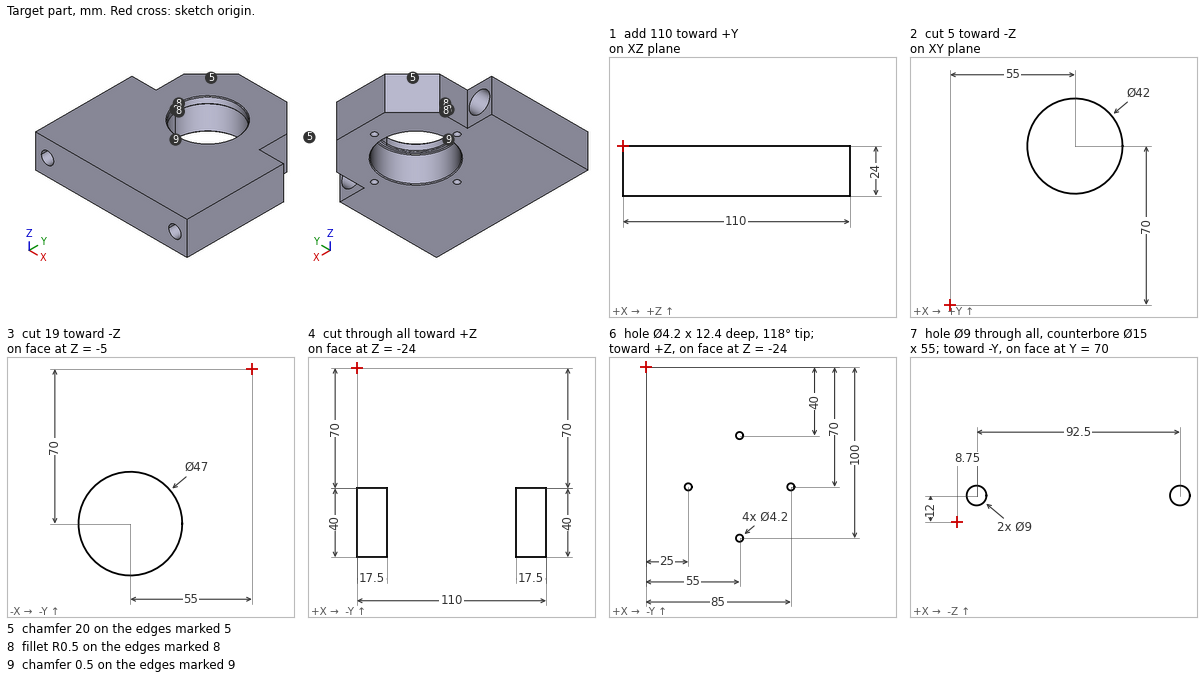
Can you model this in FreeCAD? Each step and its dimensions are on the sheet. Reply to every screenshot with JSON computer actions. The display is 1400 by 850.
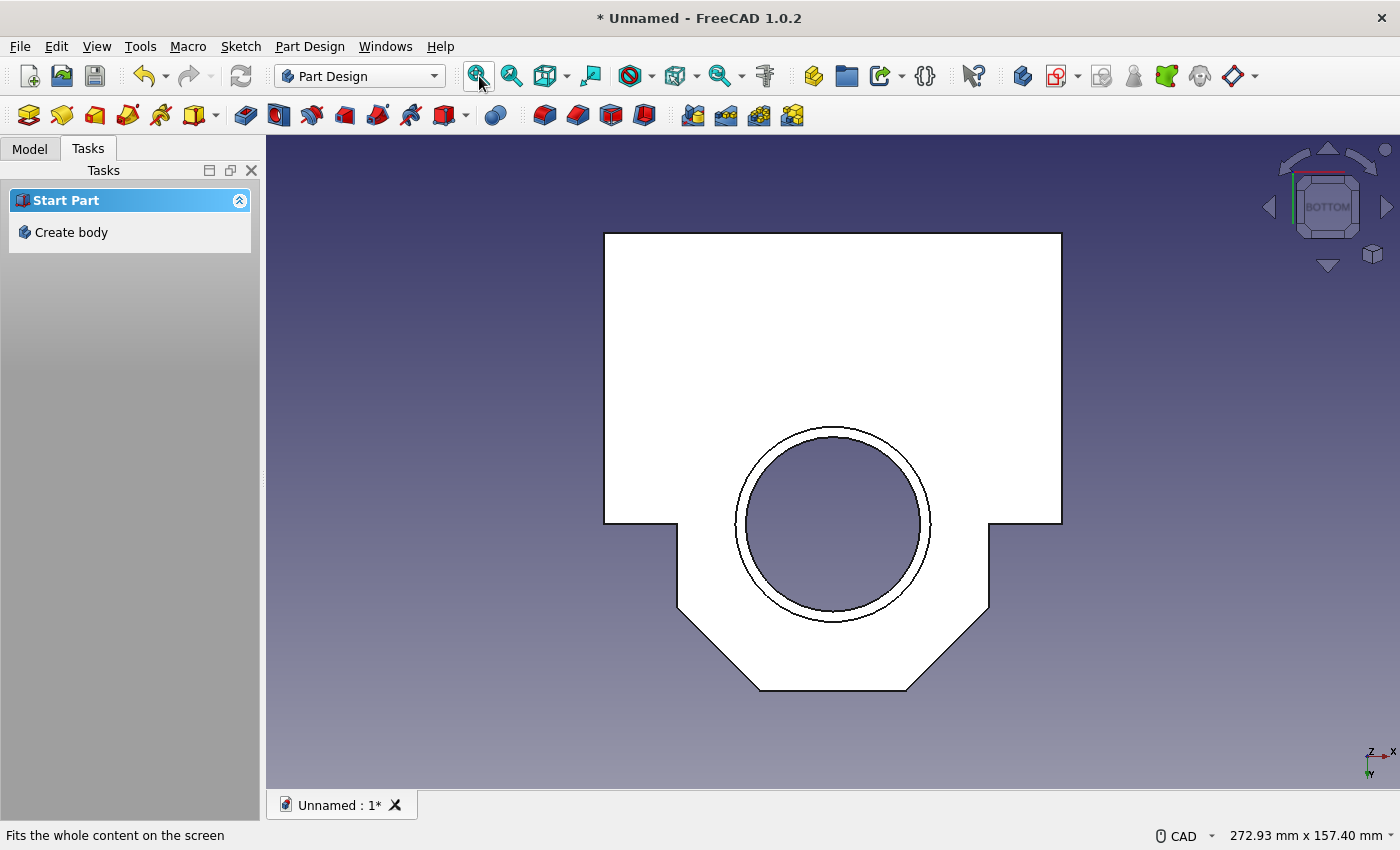
{"action": "left_click", "coordinate": [898, 330]}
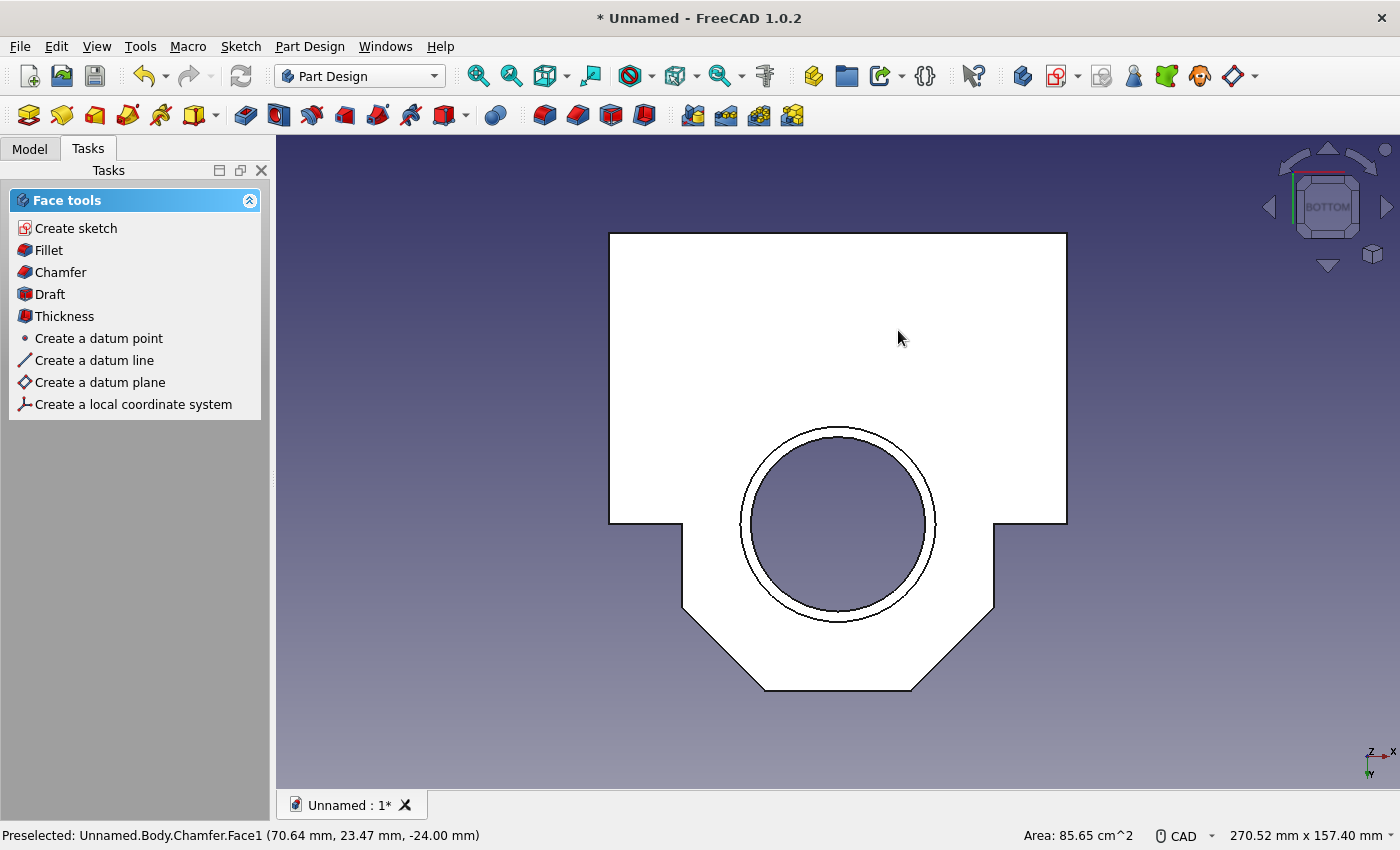
{"action": "left_click", "coordinate": [1056, 76]}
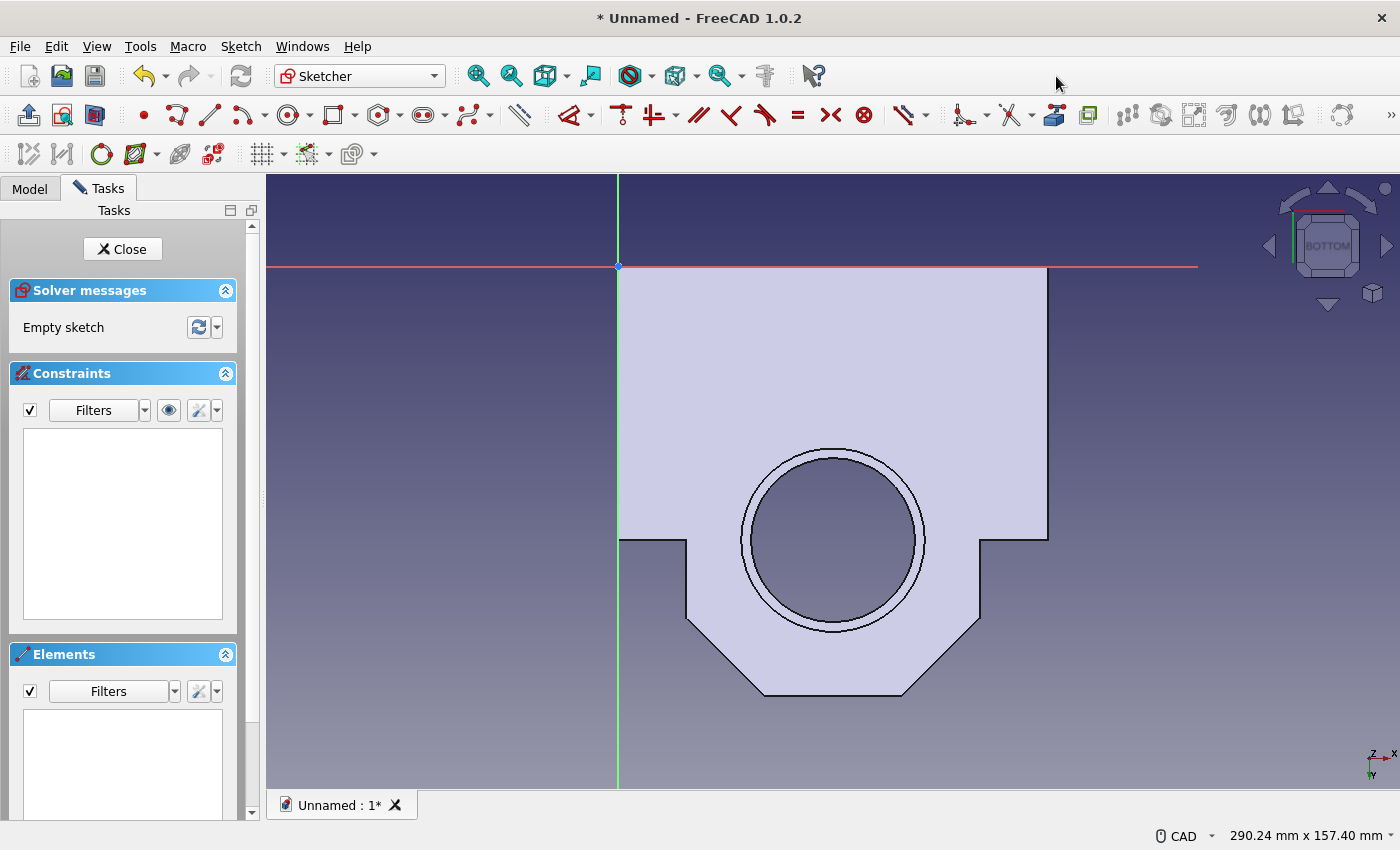
{"action": "left_click", "coordinate": [288, 116]}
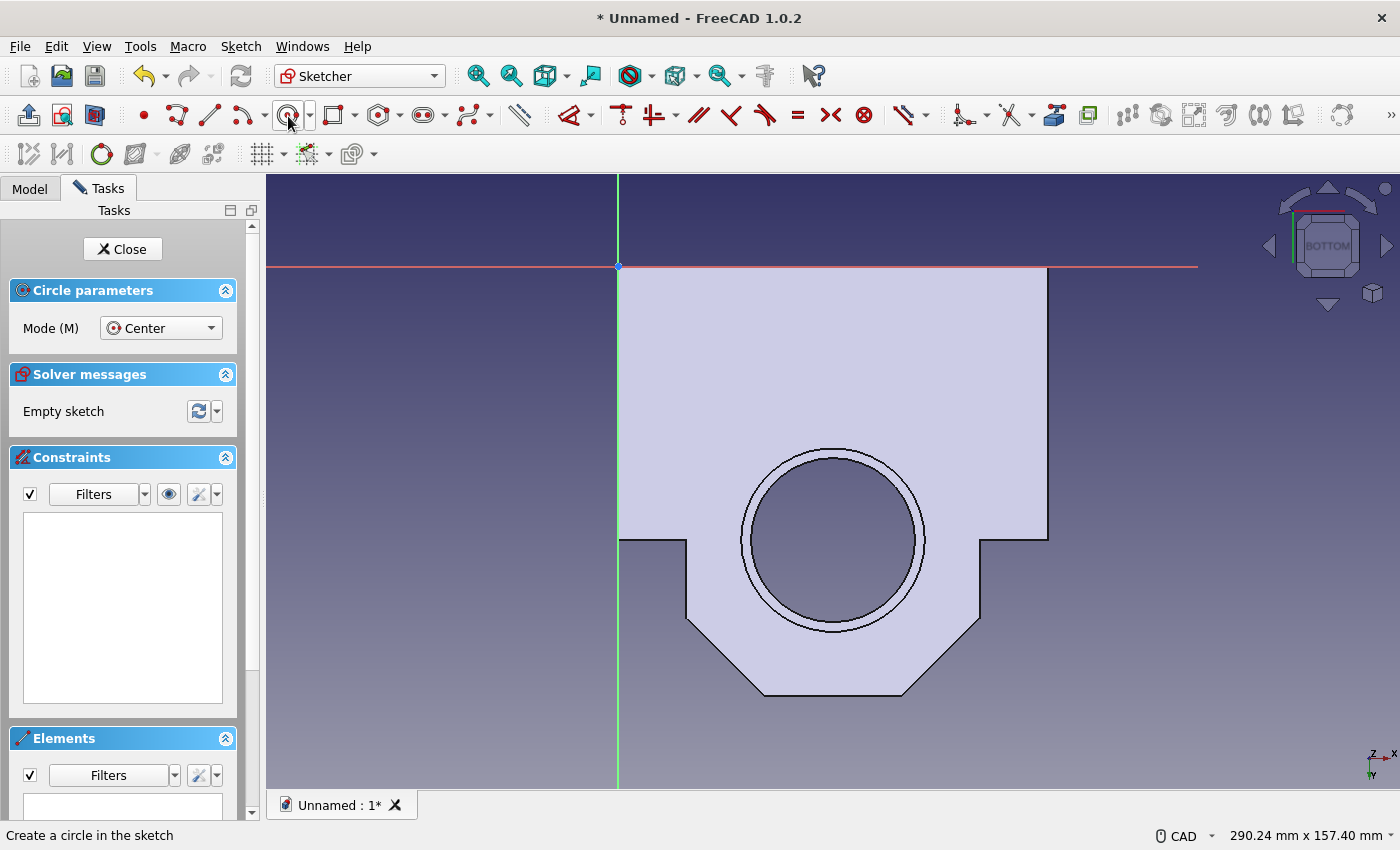
{"action": "scroll", "coordinate": [833, 657], "scroll_direction": "up", "scroll_amount": 6}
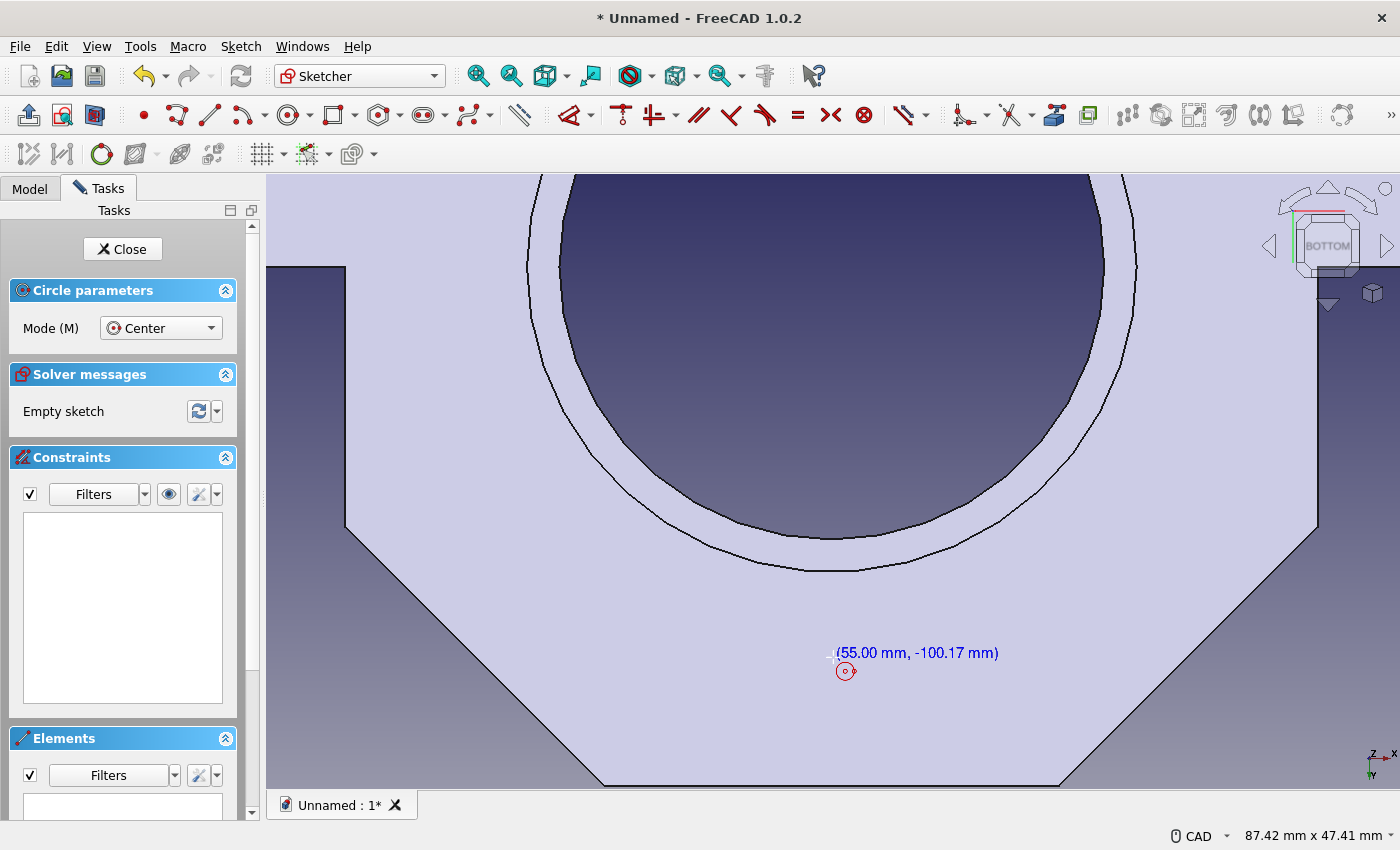
{"action": "left_click", "coordinate": [832, 656]}
{"action": "mouse_move", "coordinate": [851, 637]}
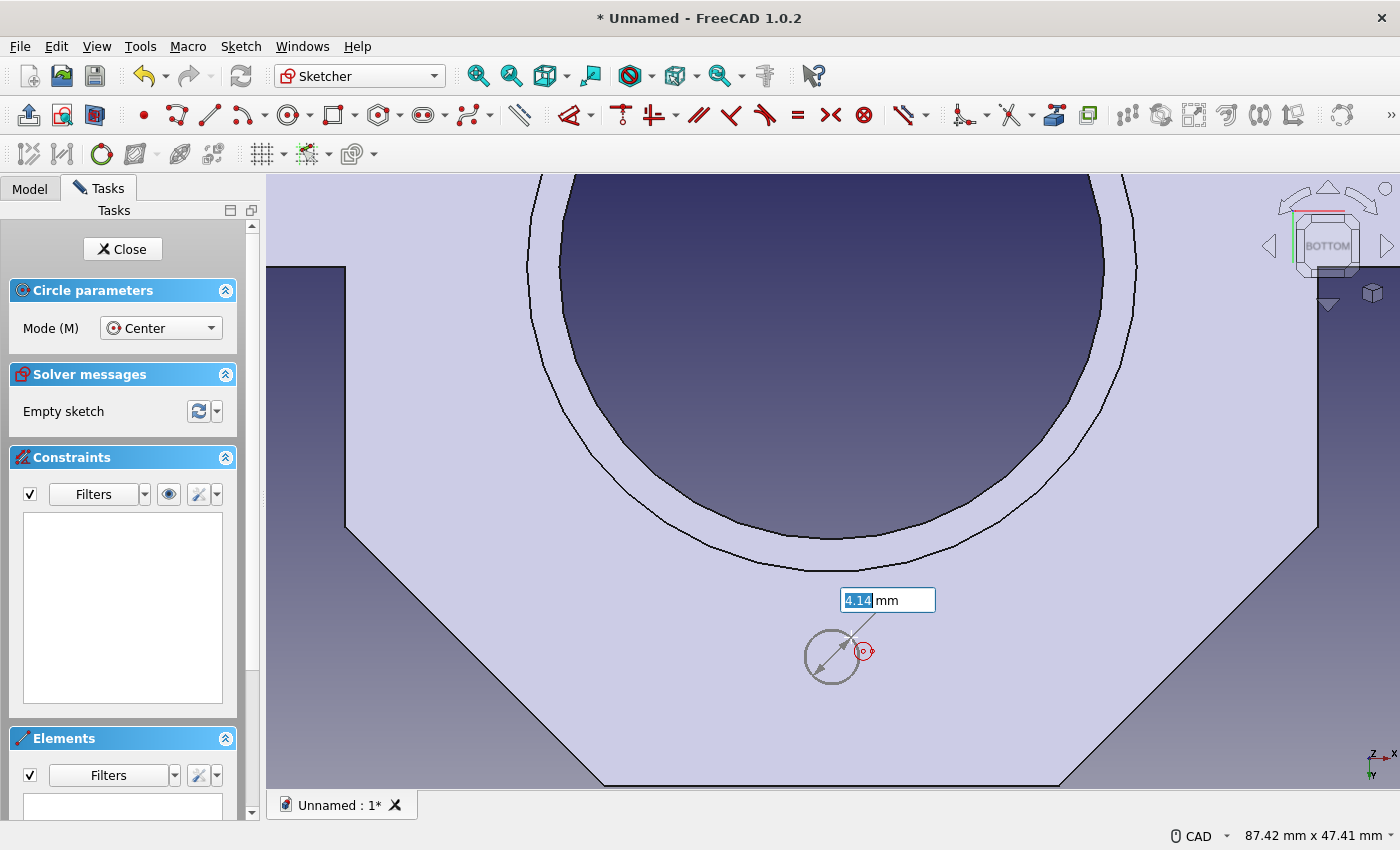
{"action": "type", "text": "4.2"}
{"action": "key", "text": "Return"}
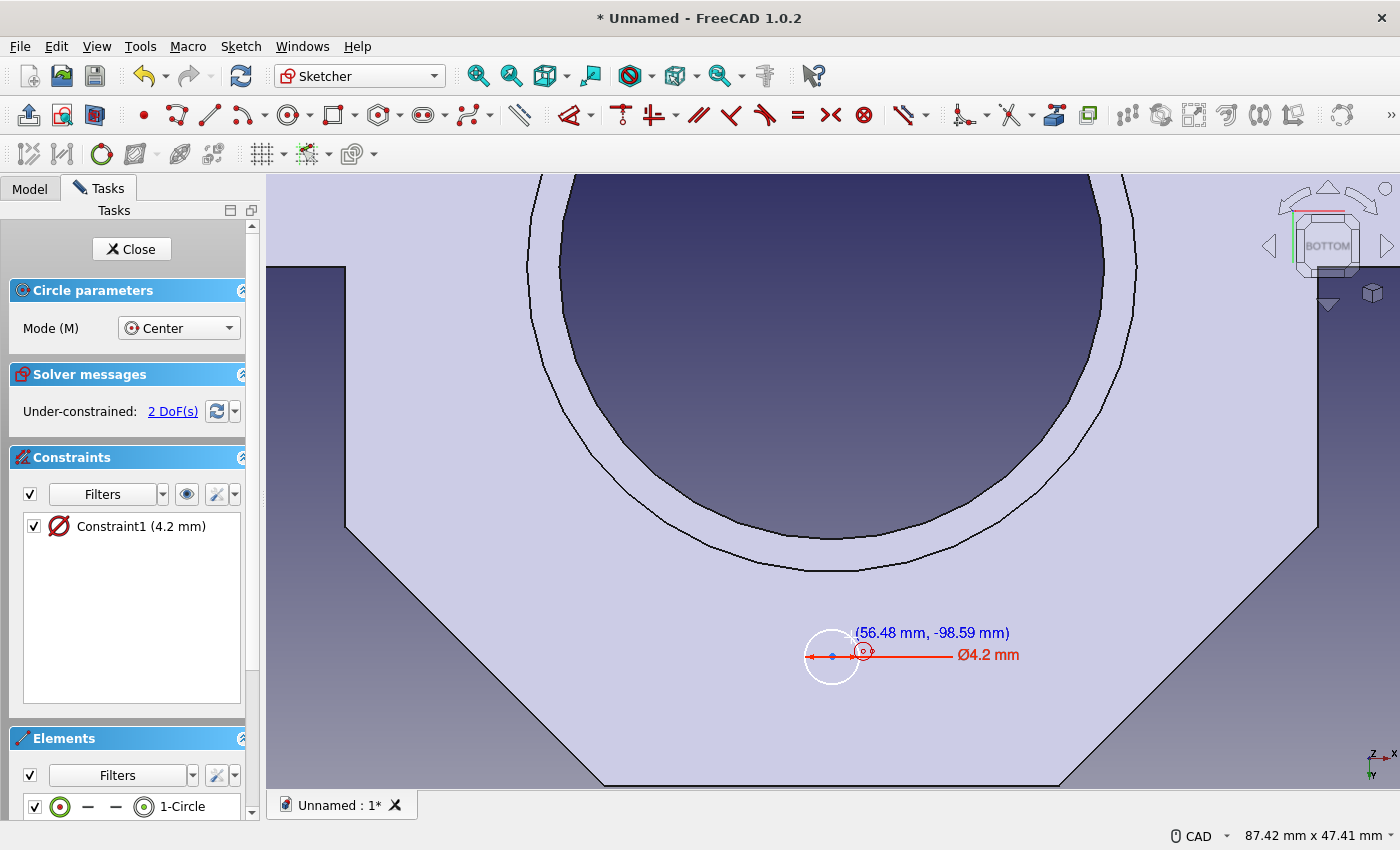
{"action": "left_click", "coordinate": [1221, 267]}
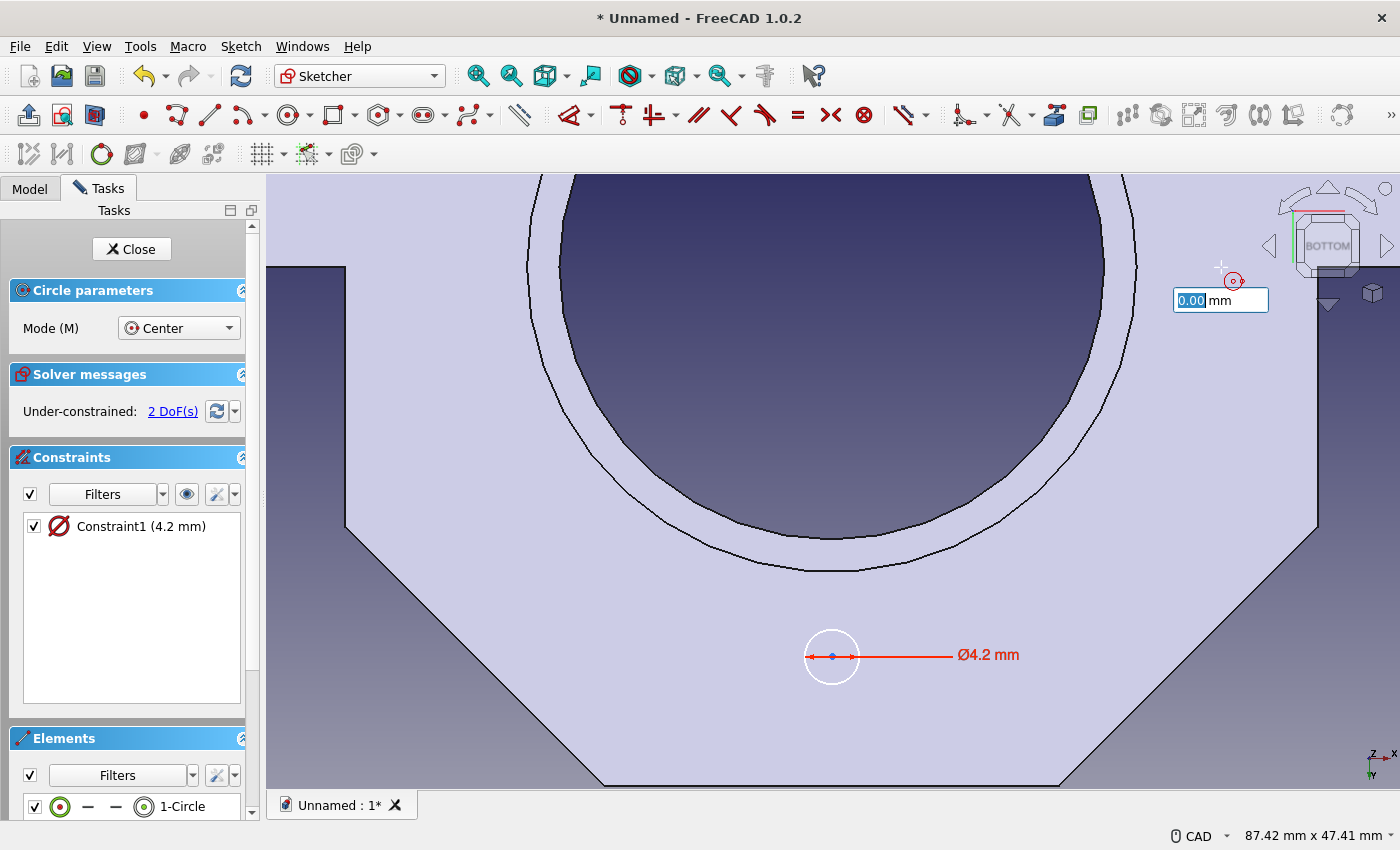
{"action": "scroll", "coordinate": [799, 680], "scroll_direction": "down", "scroll_amount": 6}
{"action": "mouse_move", "coordinate": [932, 550]}